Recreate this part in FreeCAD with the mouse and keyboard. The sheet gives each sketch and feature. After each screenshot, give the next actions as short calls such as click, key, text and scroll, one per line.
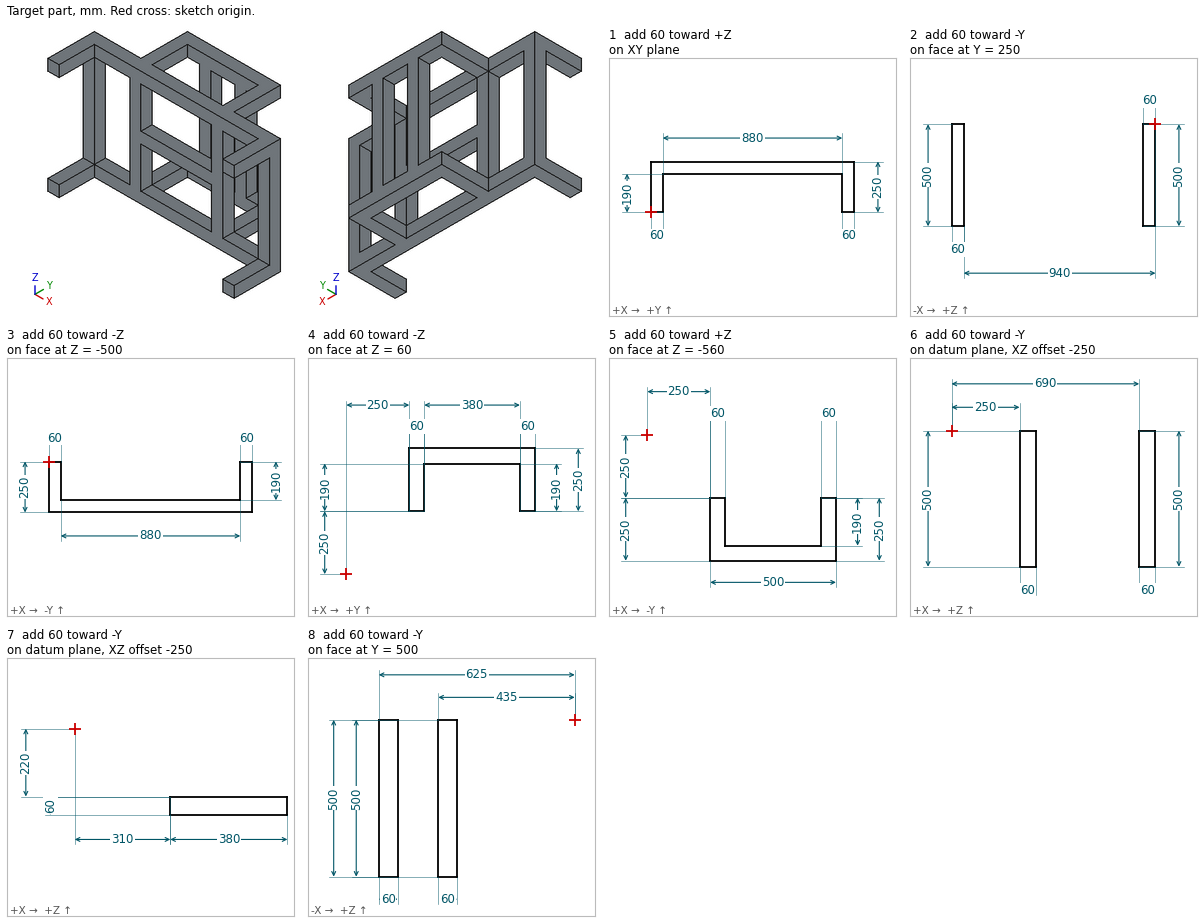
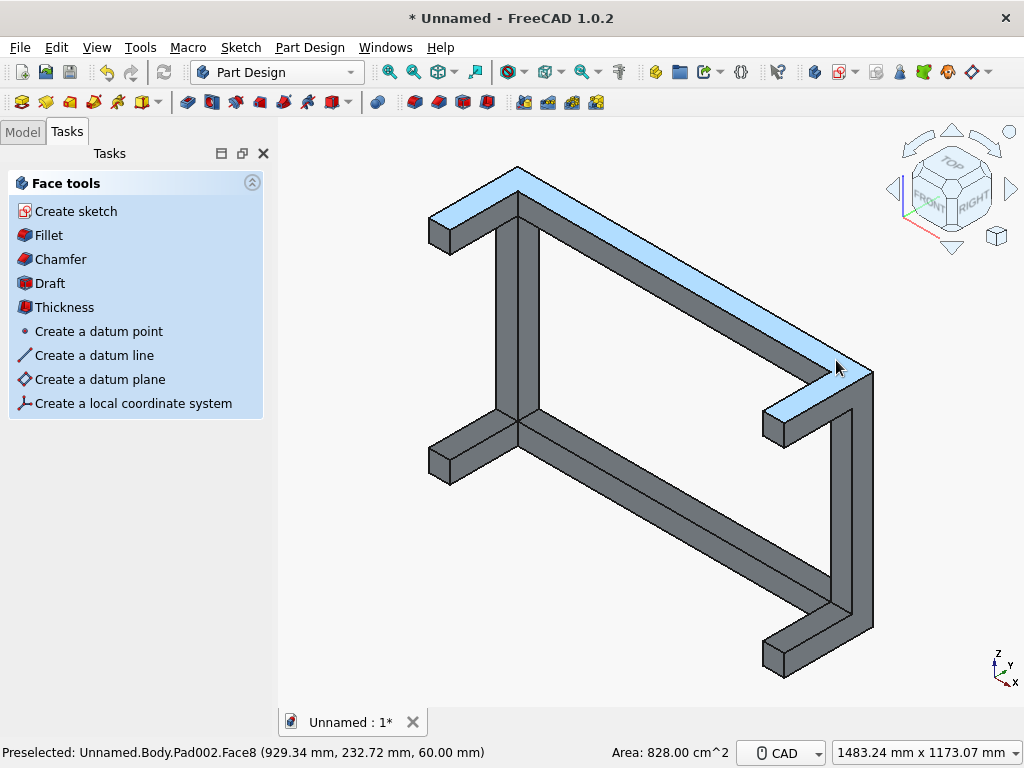
click(840, 72)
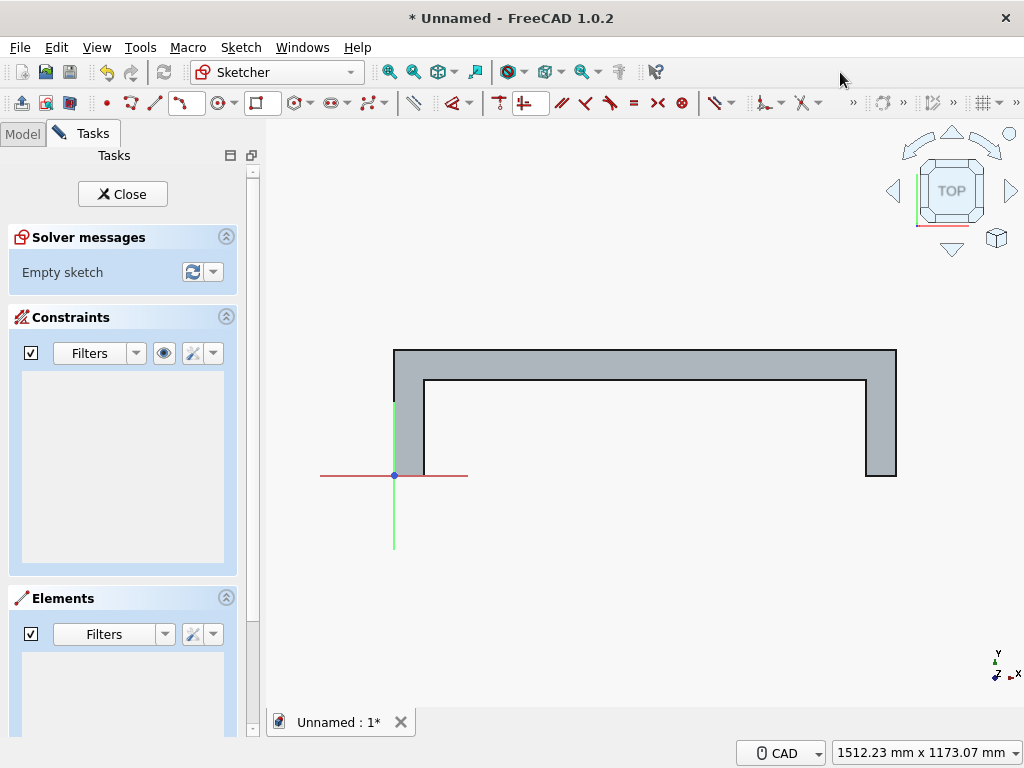
click(132, 104)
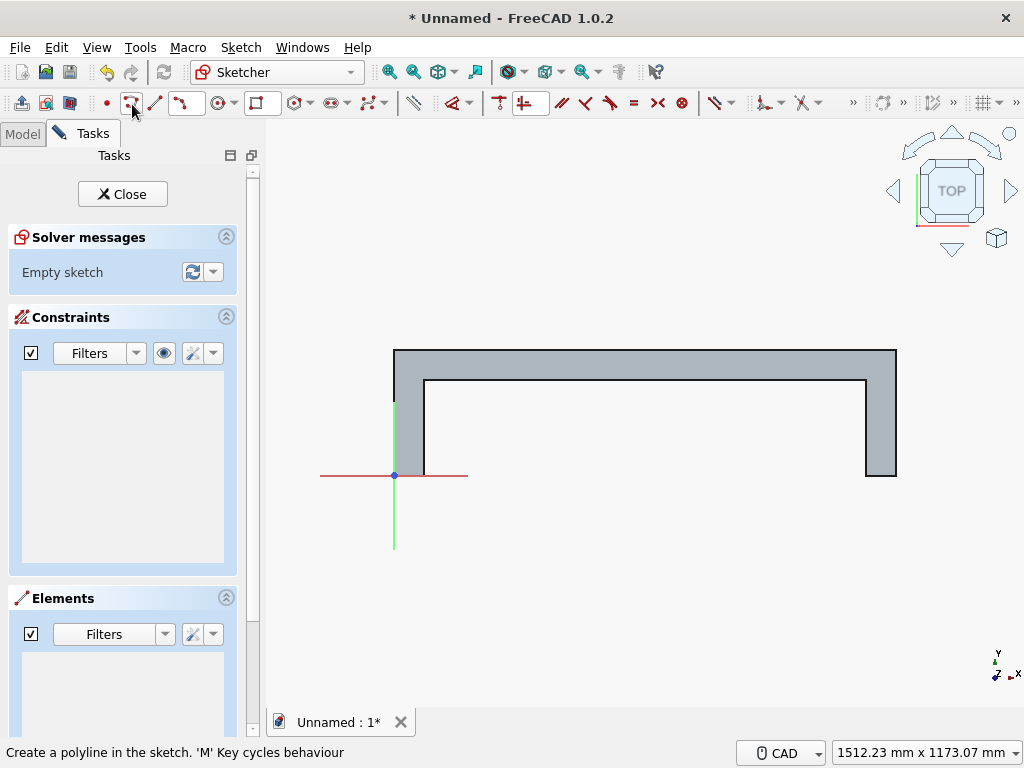
click(520, 350)
click(550, 350)
click(550, 255)
click(740, 255)
click(740, 350)
click(770, 350)
click(770, 225)
click(520, 225)
click(520, 351)
key(Escape)
key(Escape)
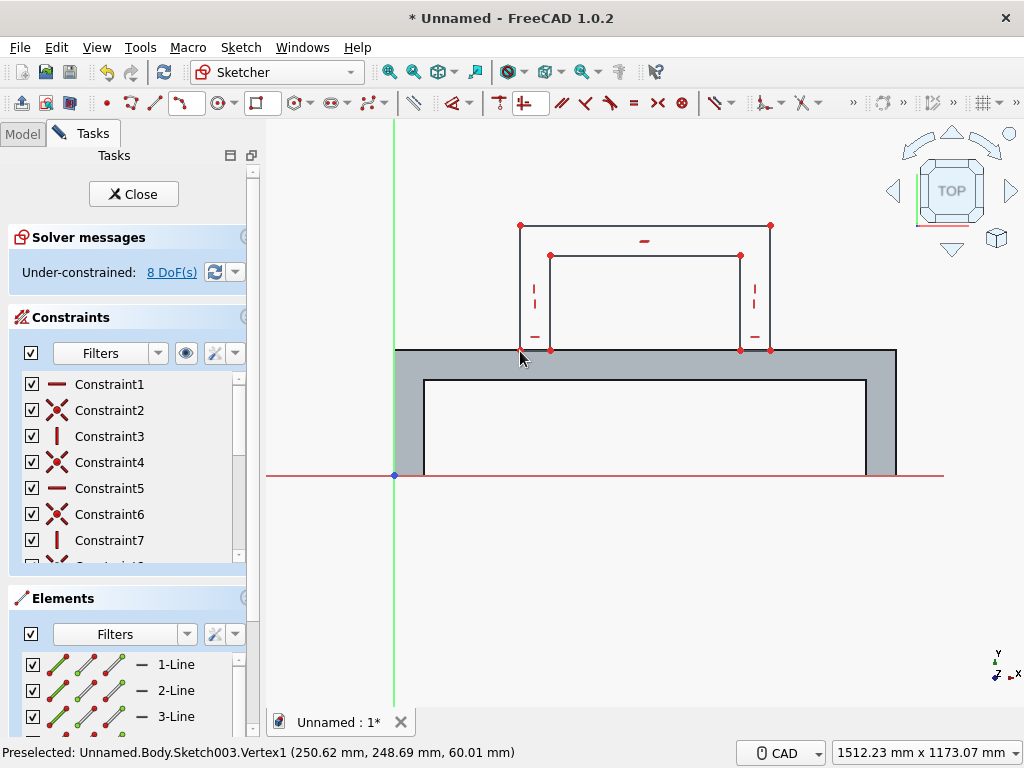
click(452, 104)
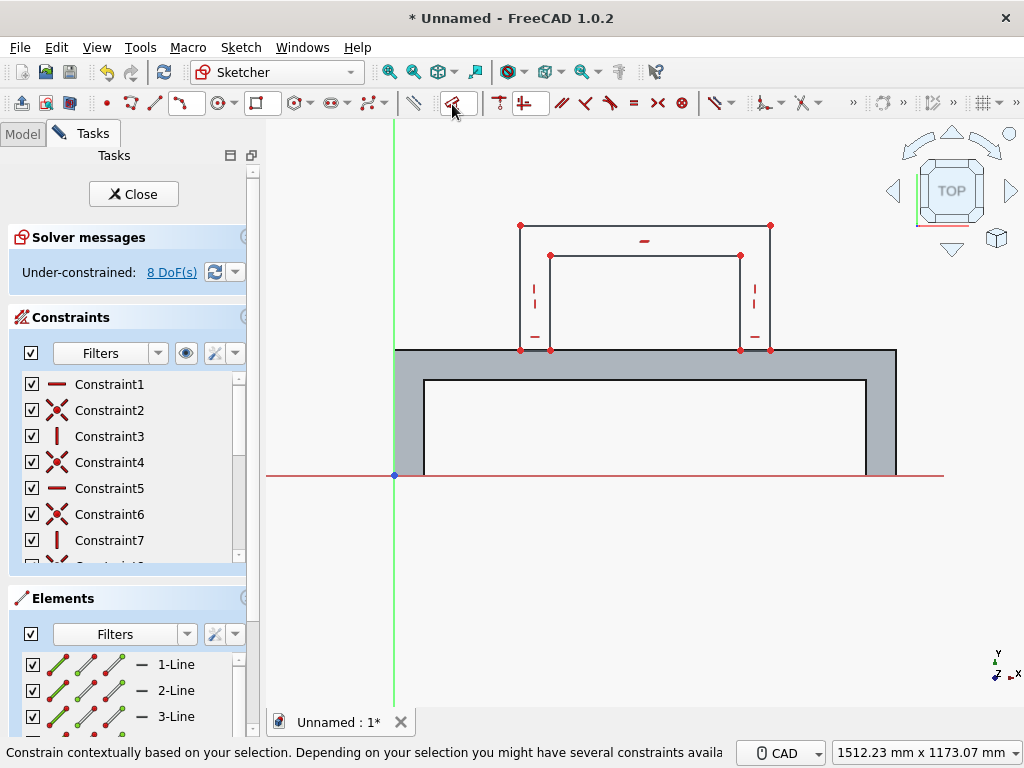
scroll(532, 351, up, 2)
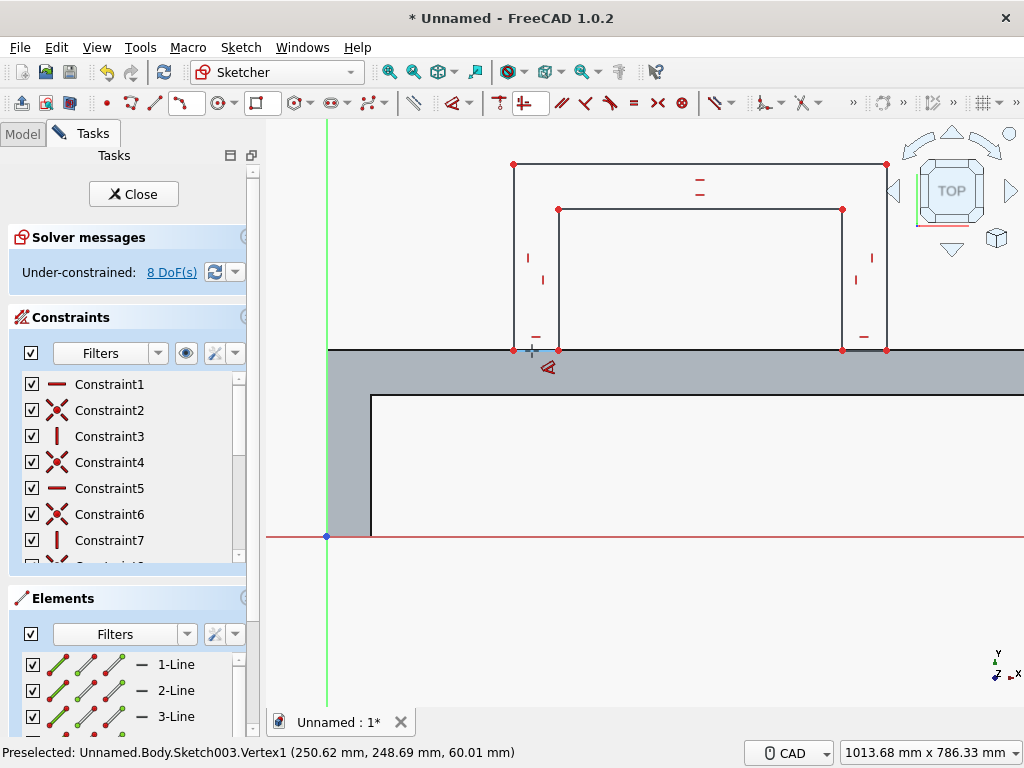
click(532, 351)
click(536, 385)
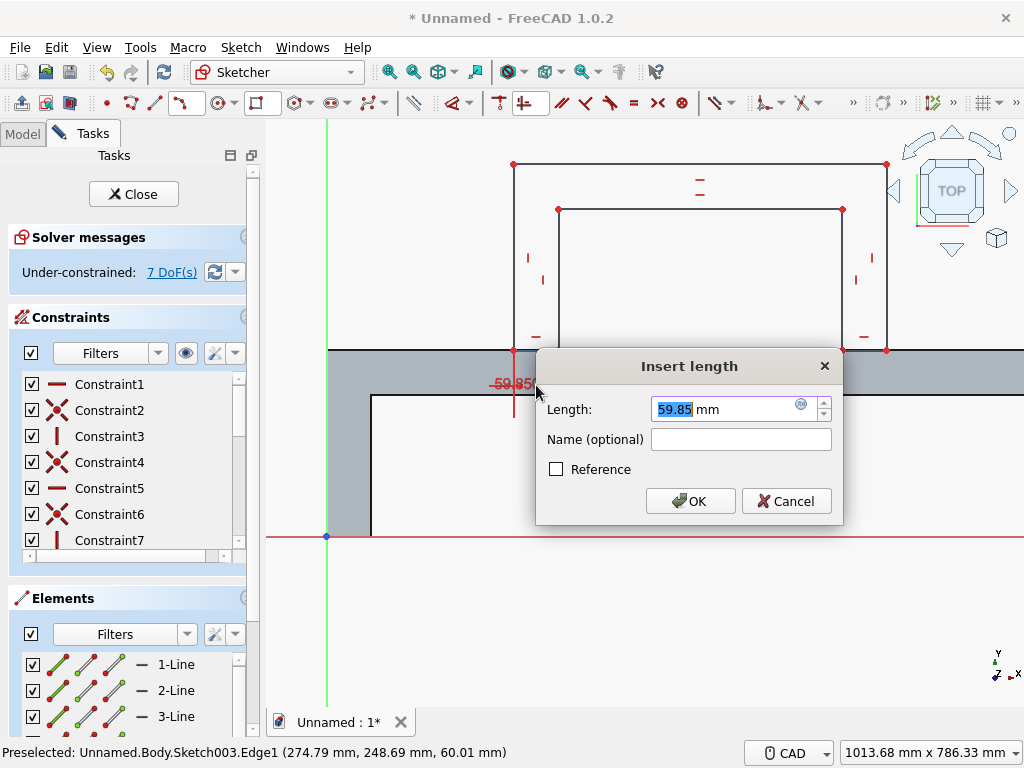
text(60)
key(Return)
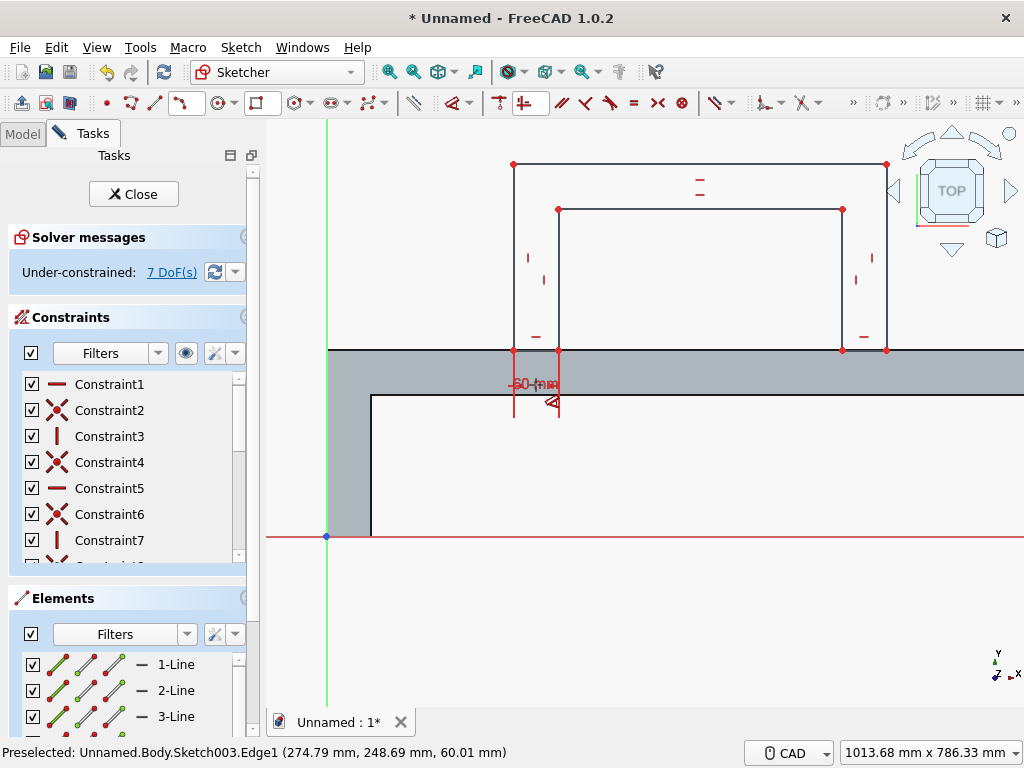
click(856, 351)
click(851, 385)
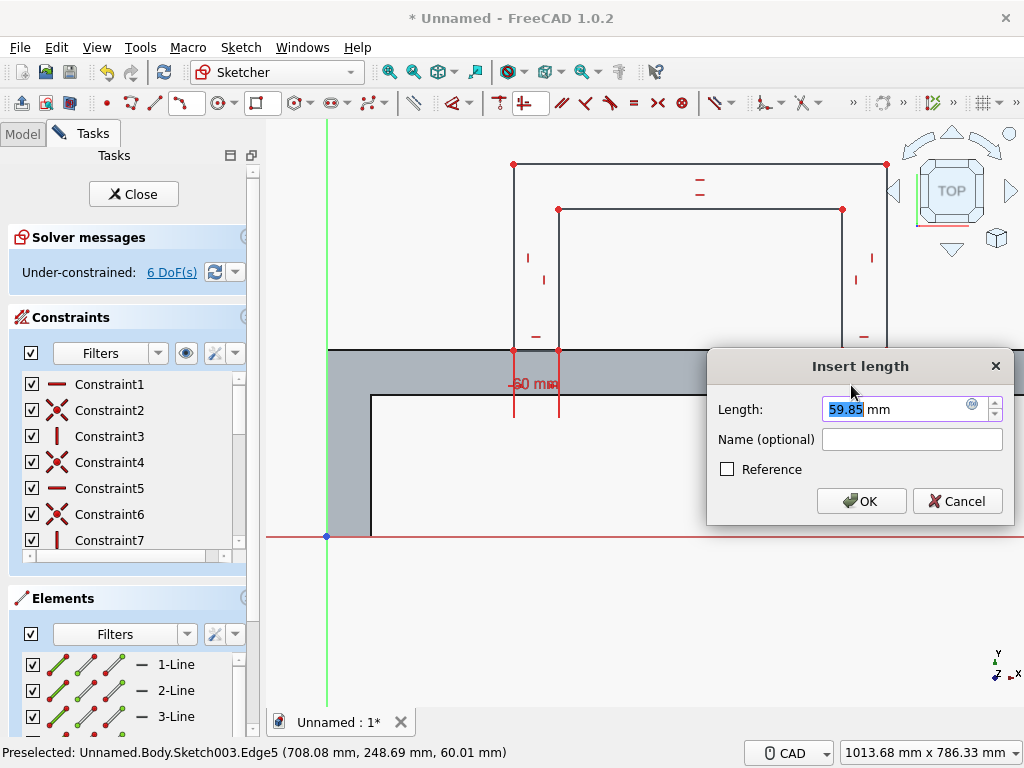
text(60)
key(Return)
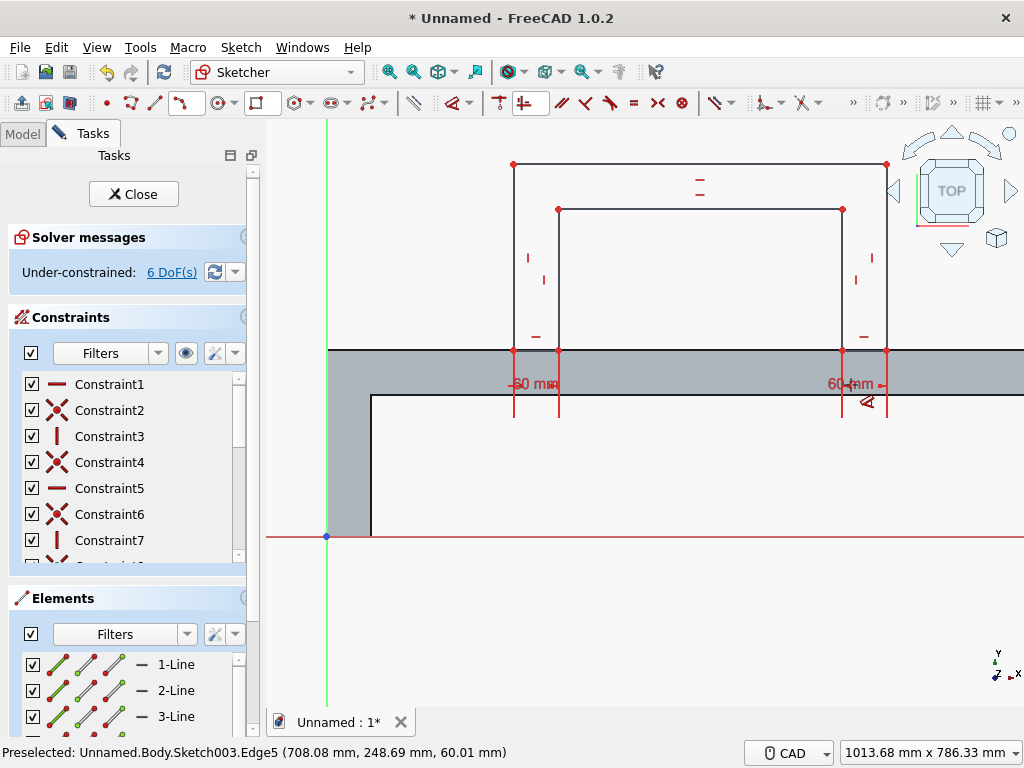
click(559, 308)
click(593, 280)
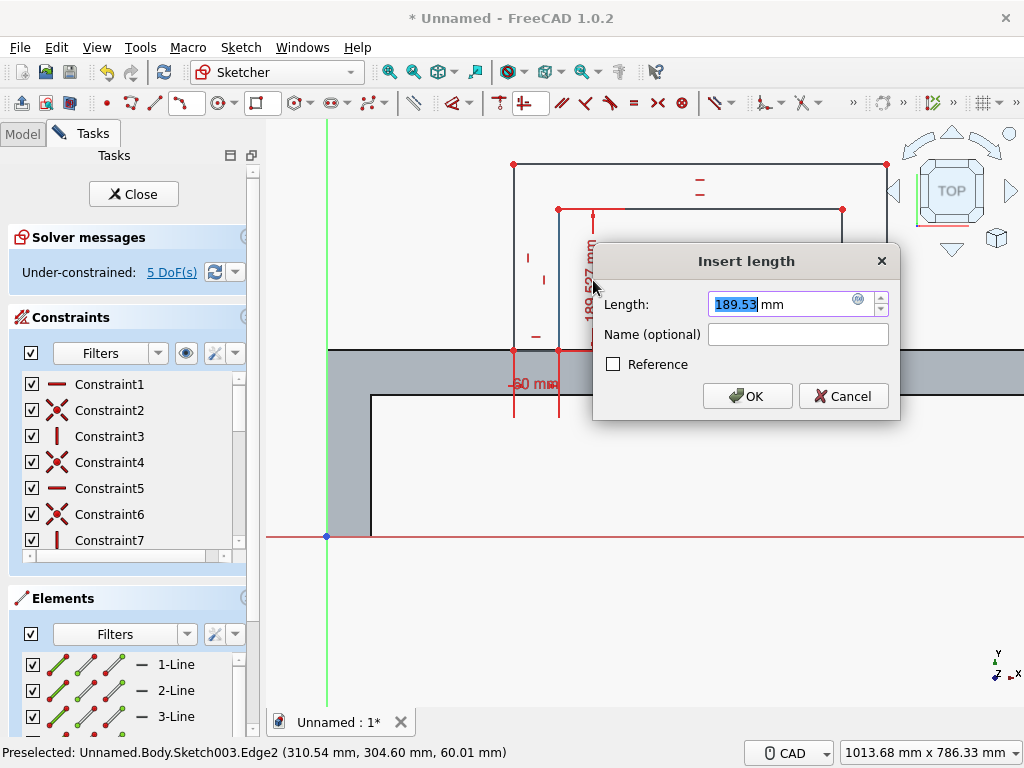
text(190)
key(Return)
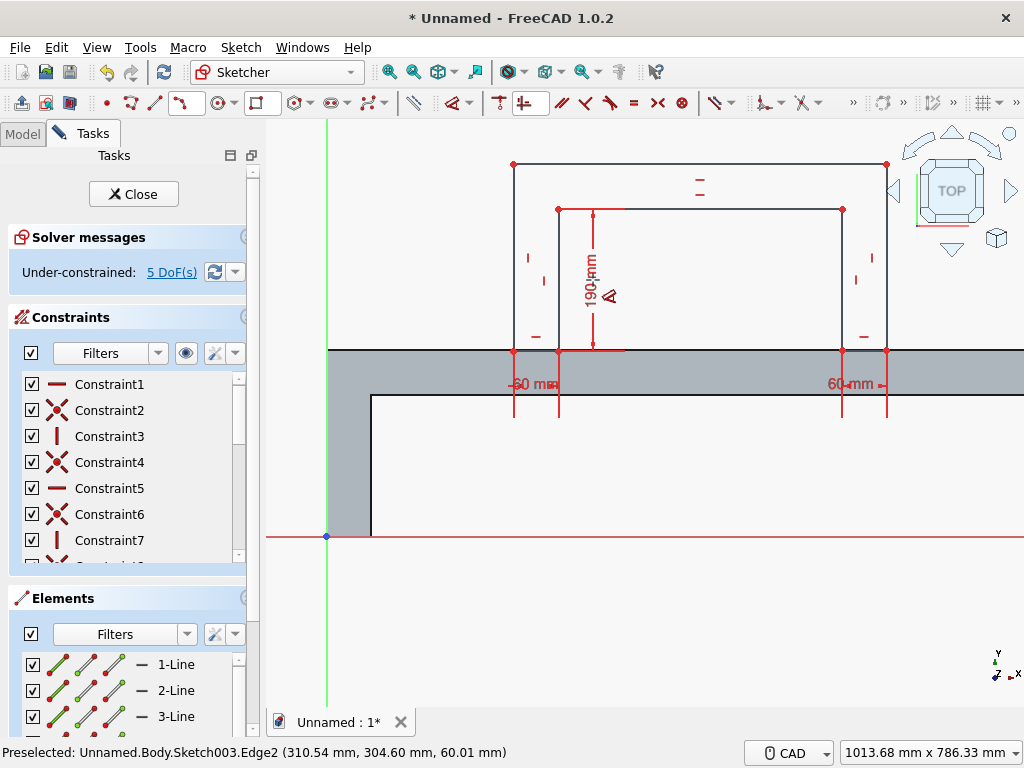
click(644, 209)
click(700, 243)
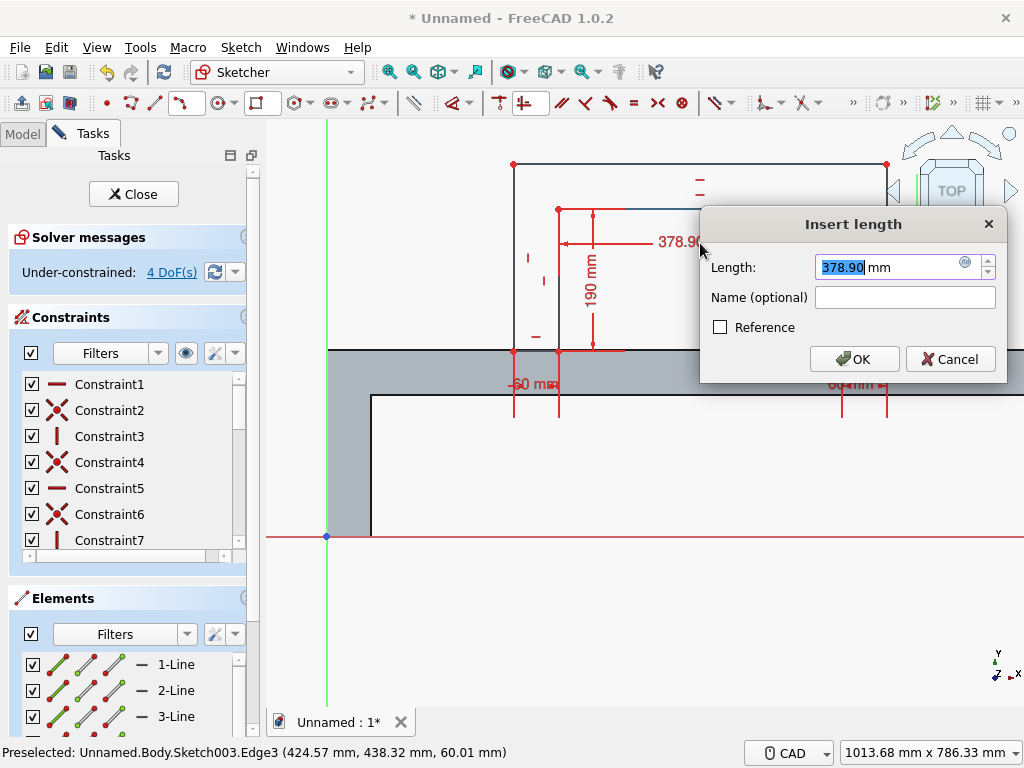
text(380)
key(Return)